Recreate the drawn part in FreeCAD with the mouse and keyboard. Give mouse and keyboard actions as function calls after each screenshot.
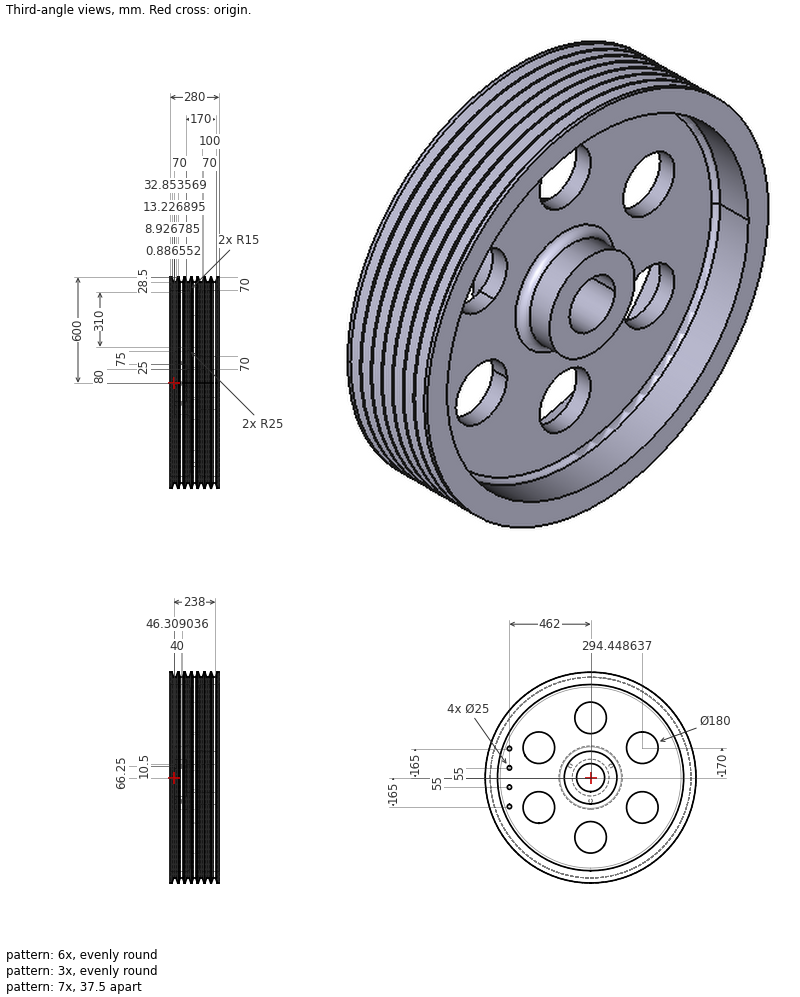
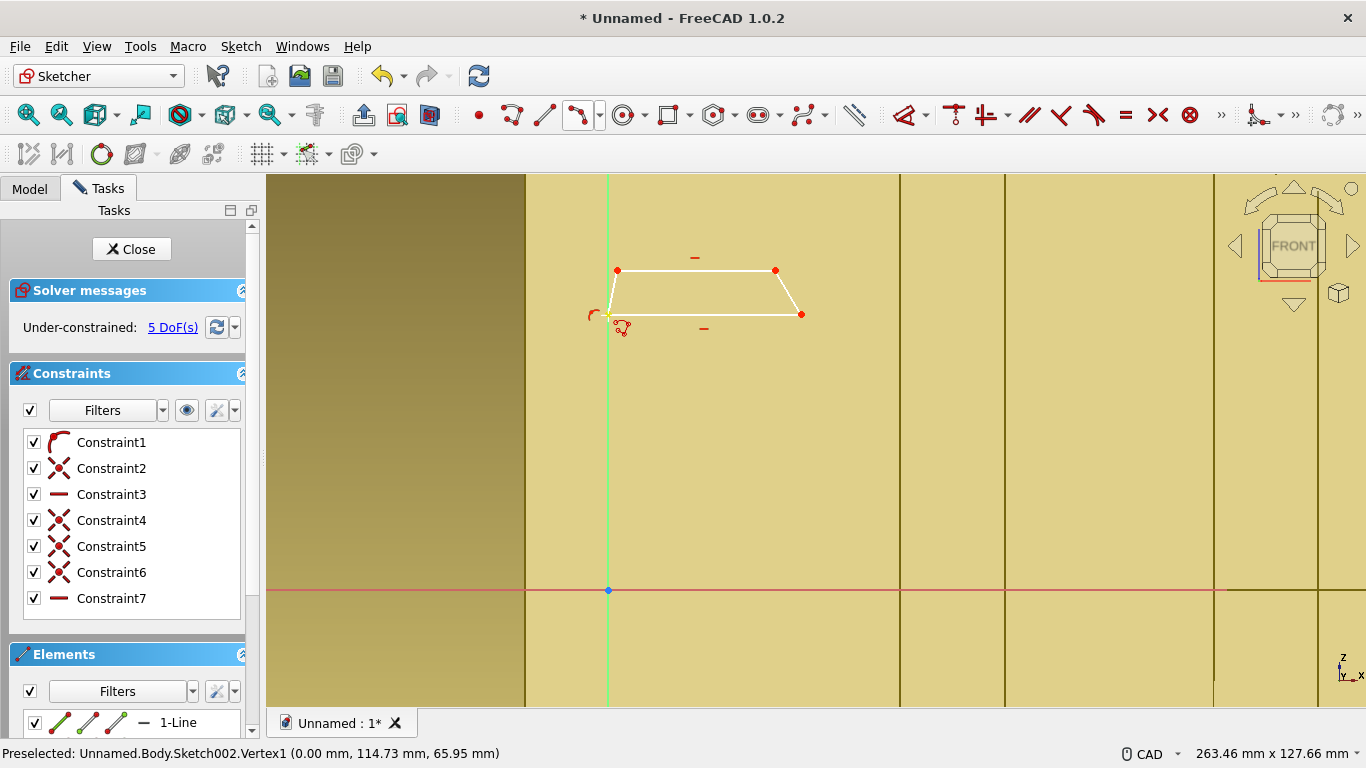
click(545, 116)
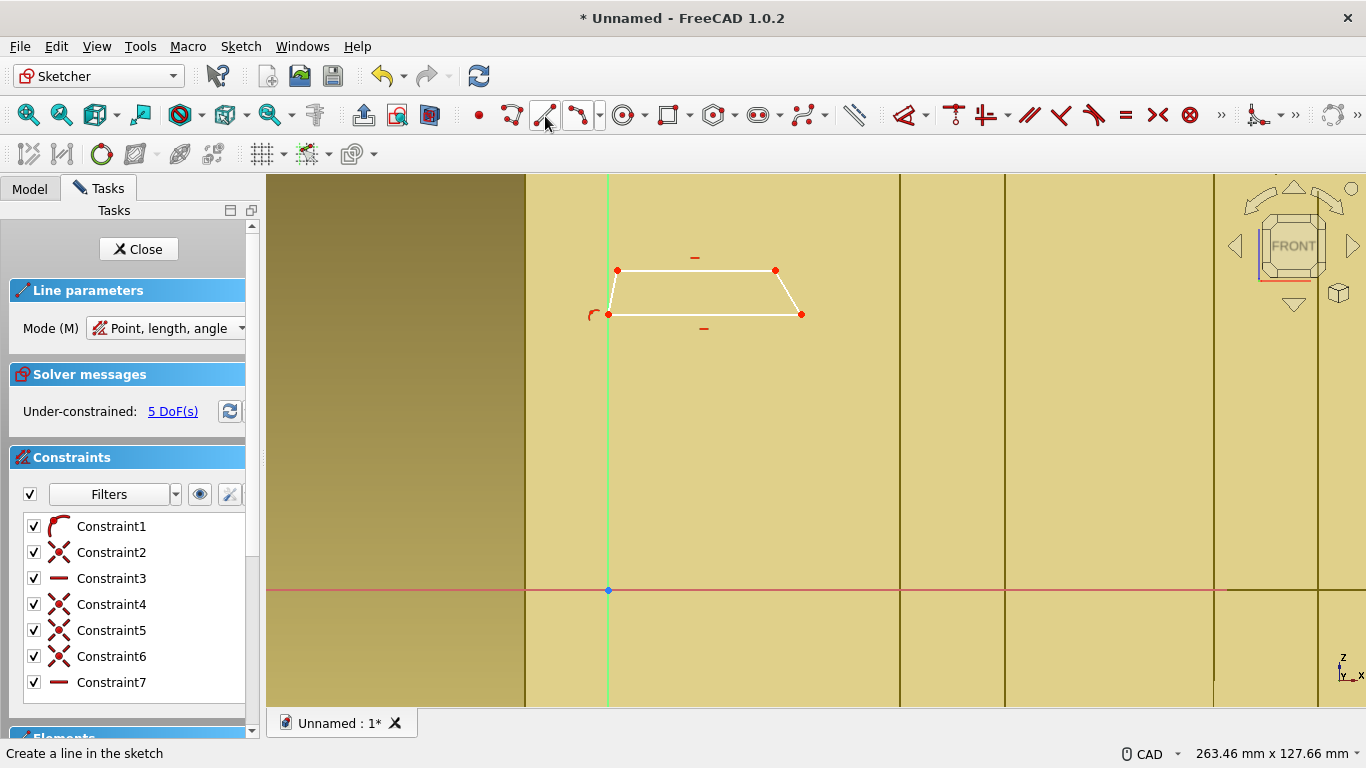
click(821, 314)
click(879, 314)
key(Escape)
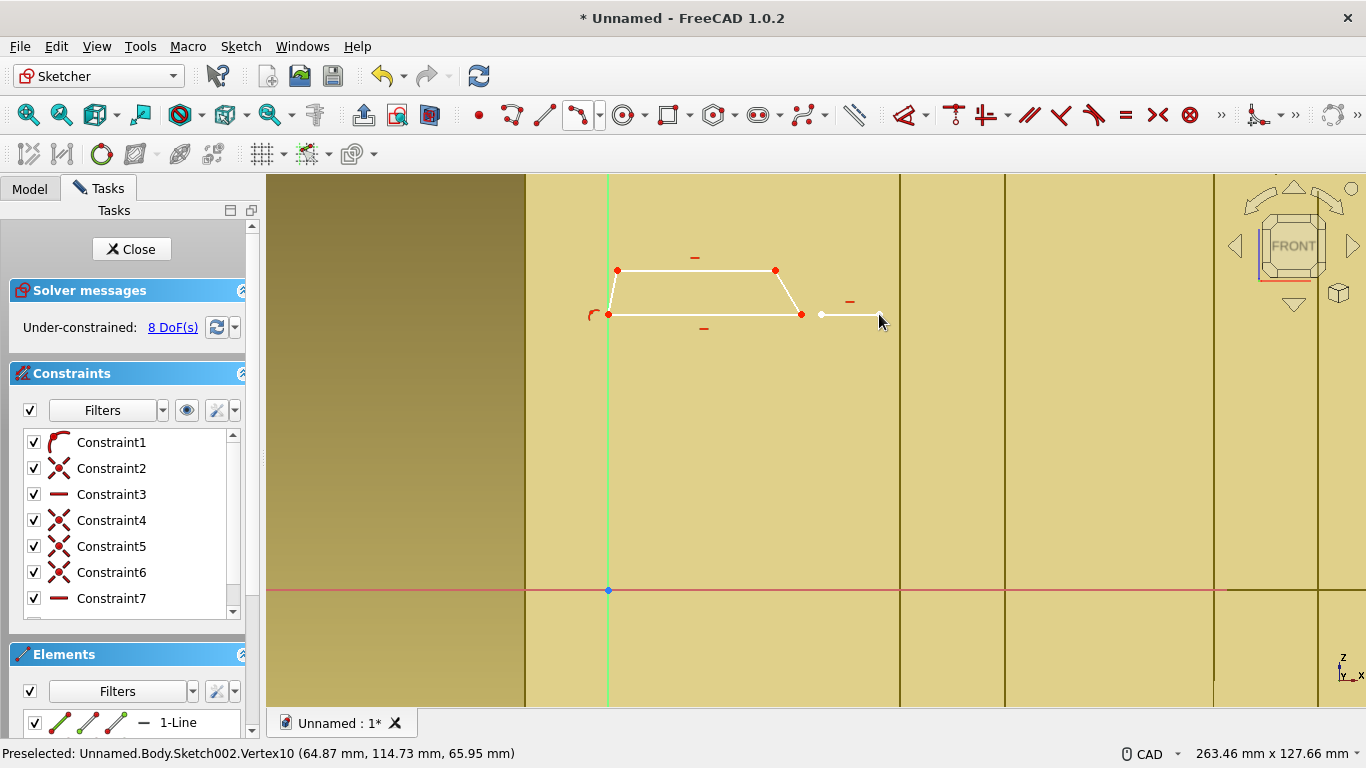
click(838, 315)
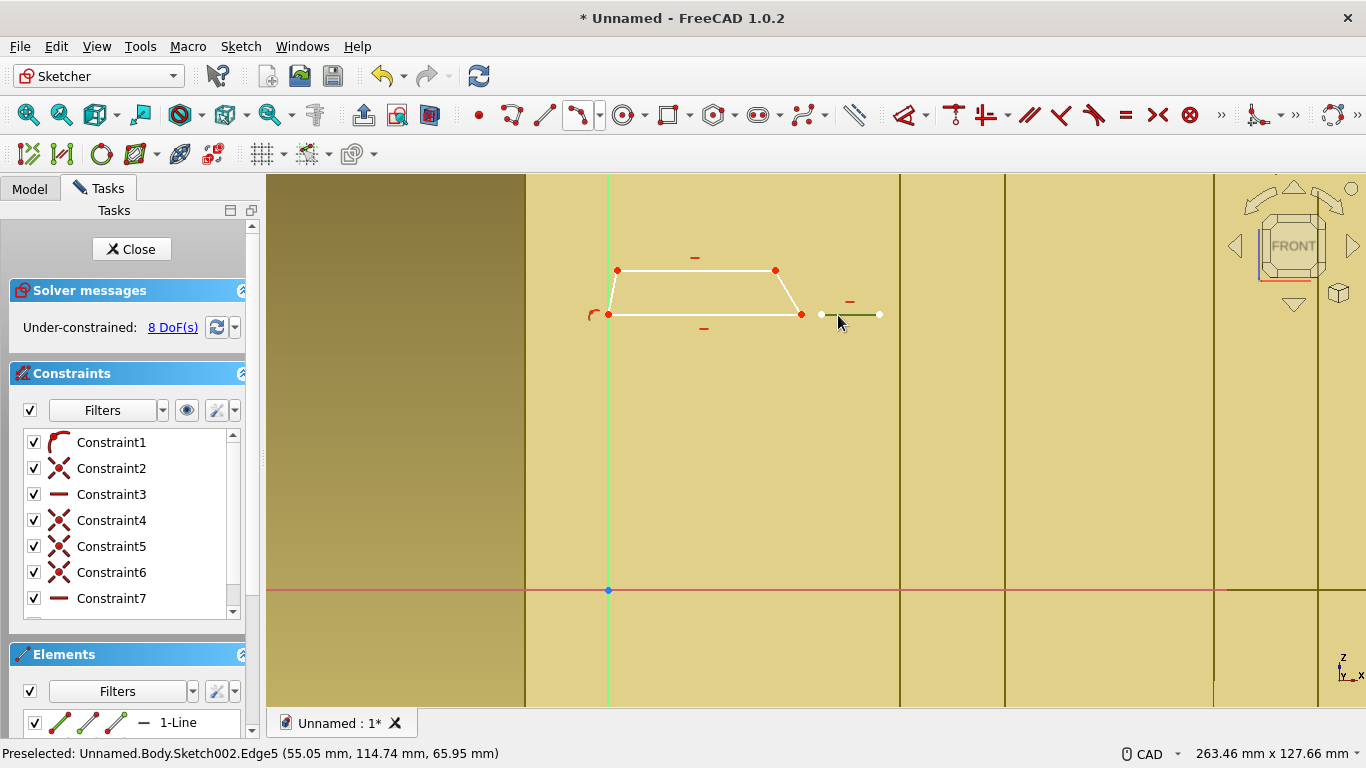
click(855, 116)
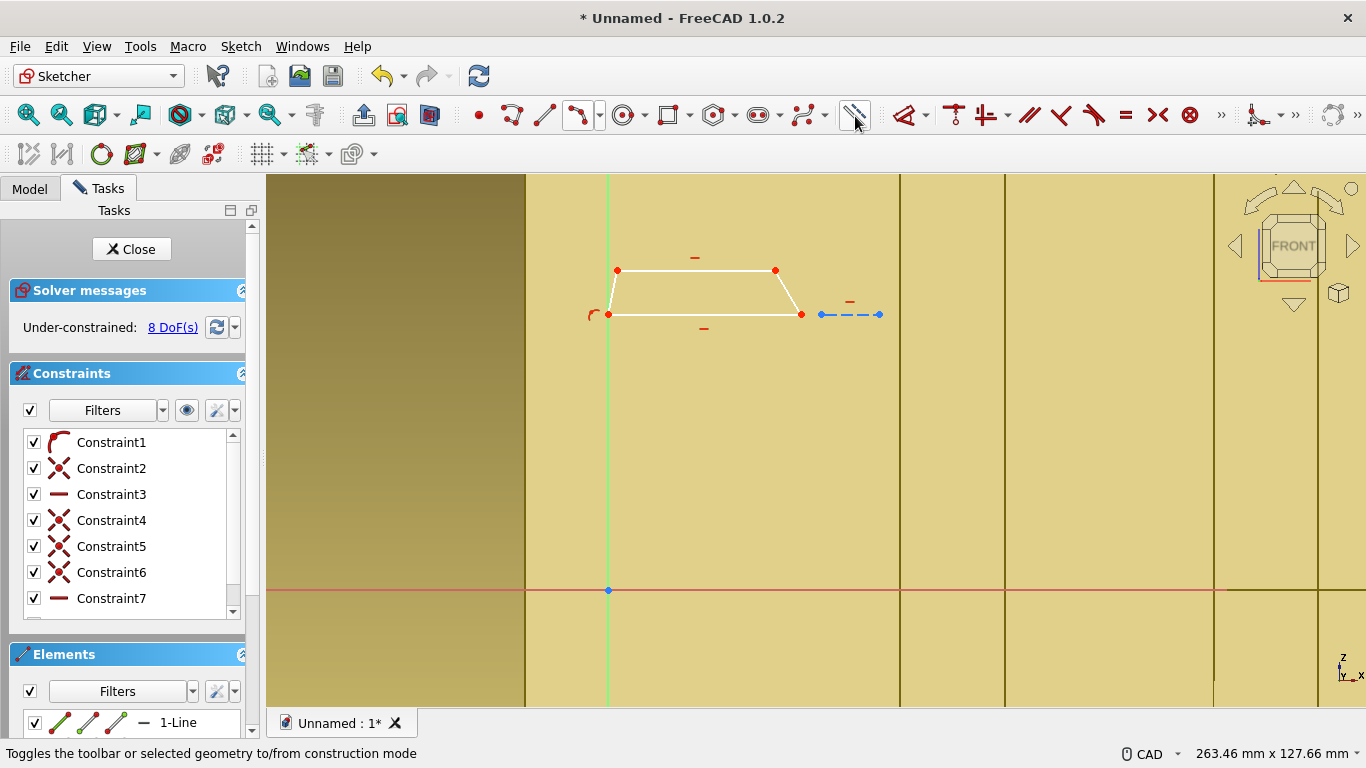
click(611, 302)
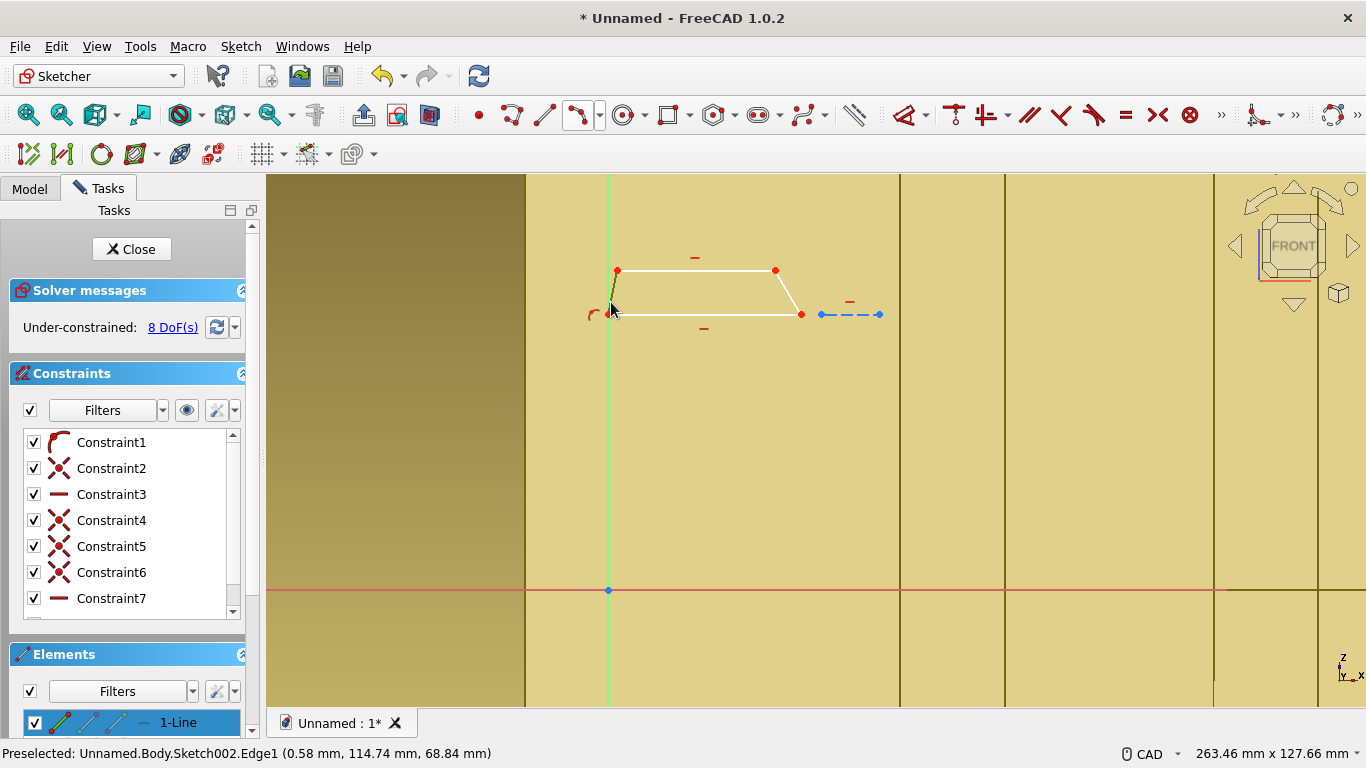
click(1008, 116)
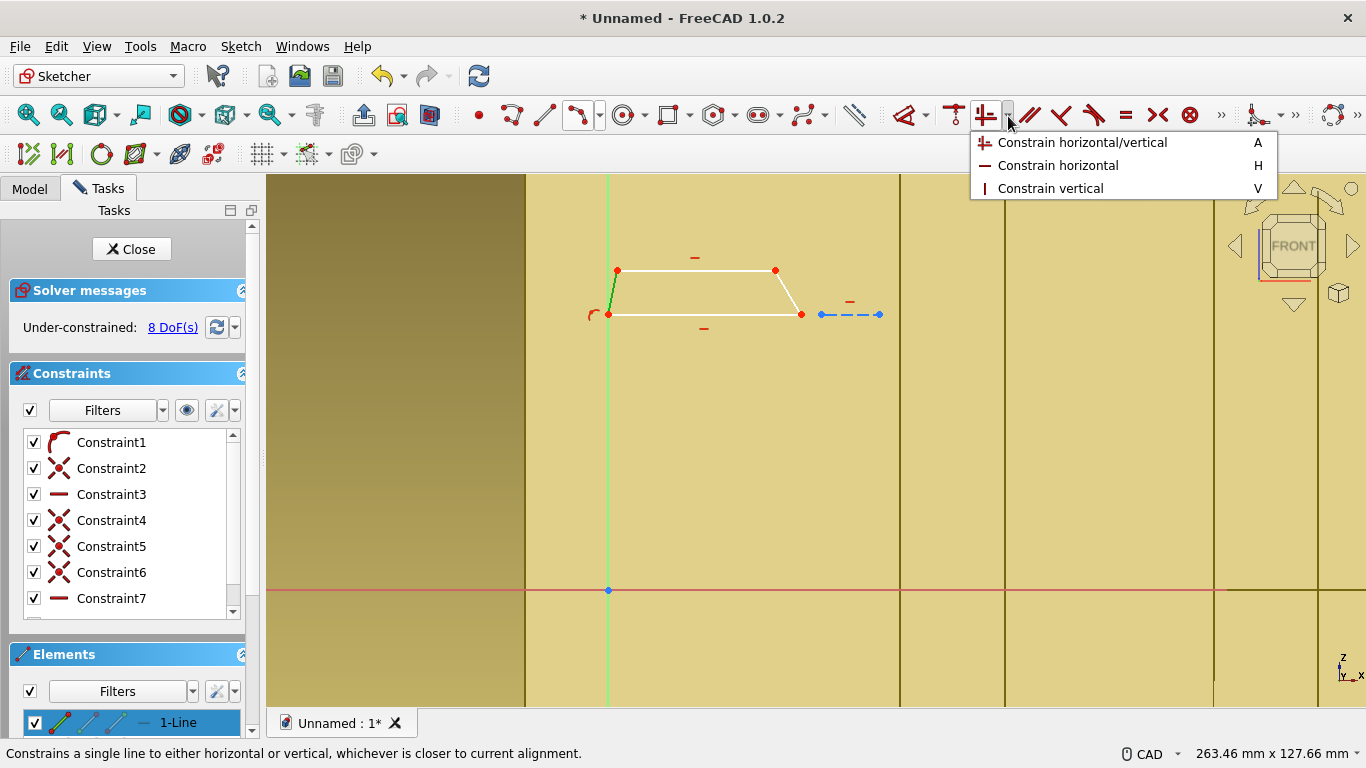
click(1124, 188)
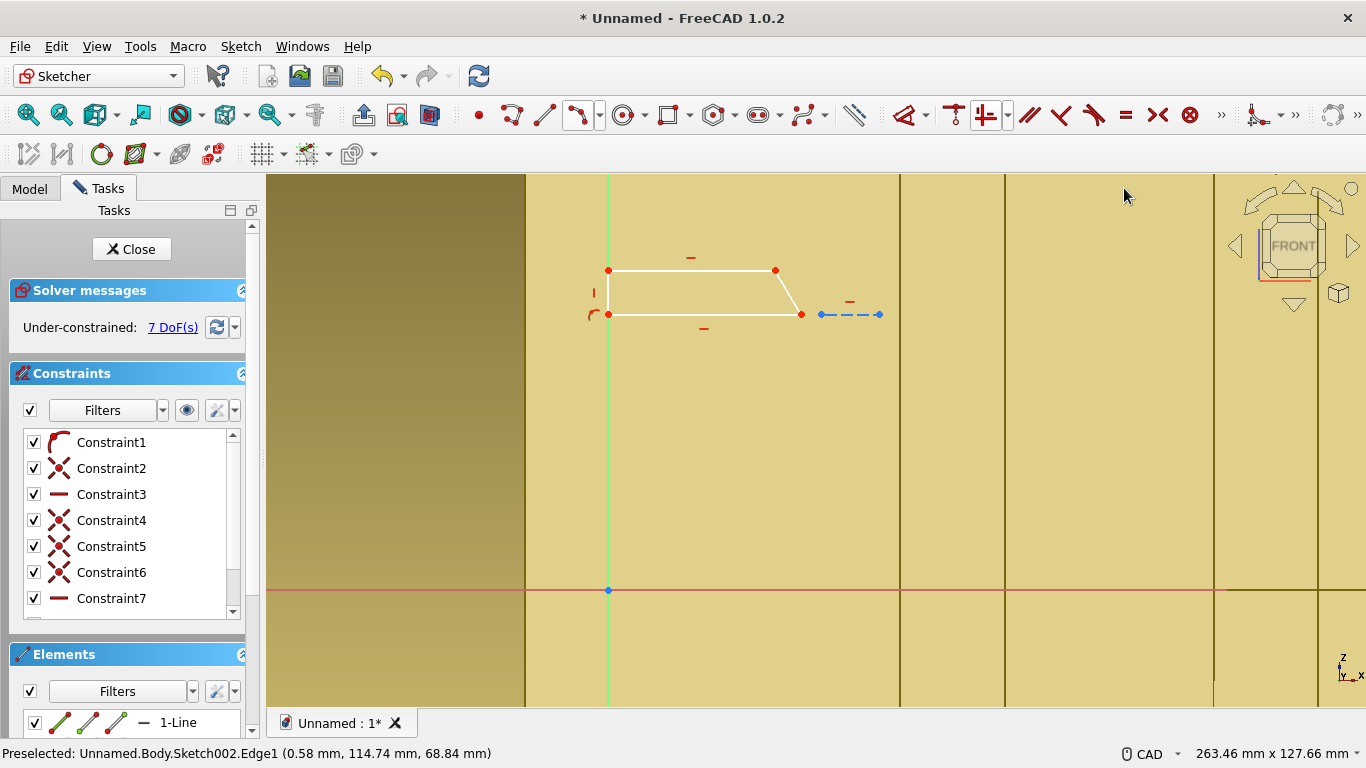
click(904, 116)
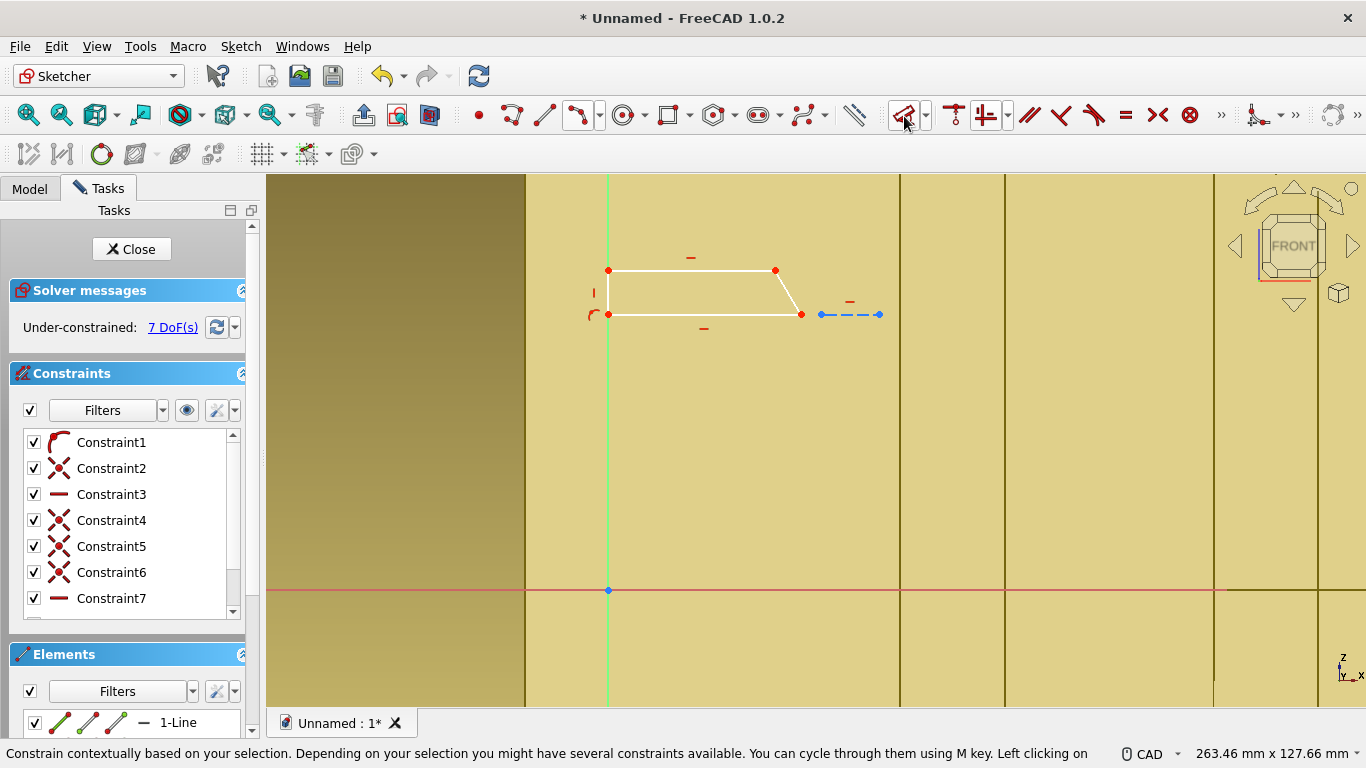
click(658, 271)
click(692, 237)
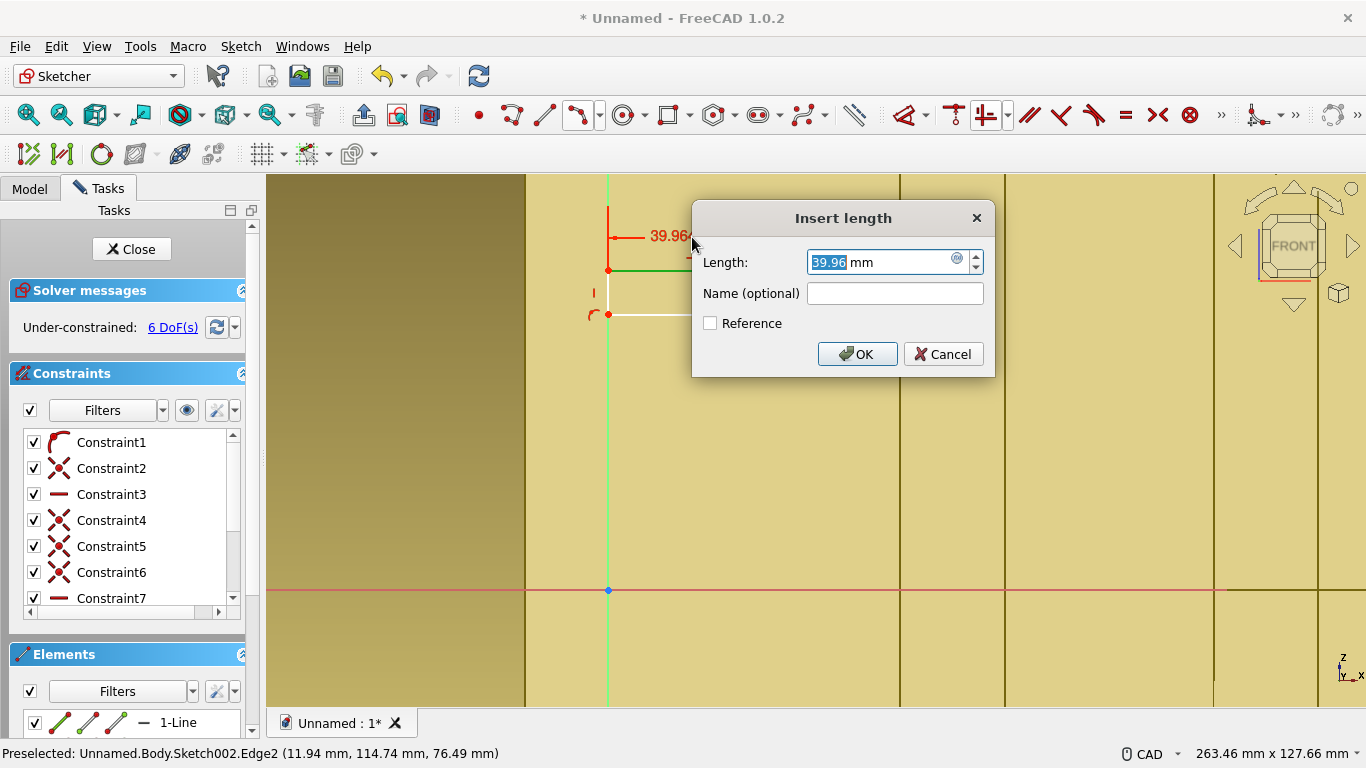
text(40)
key(Return)